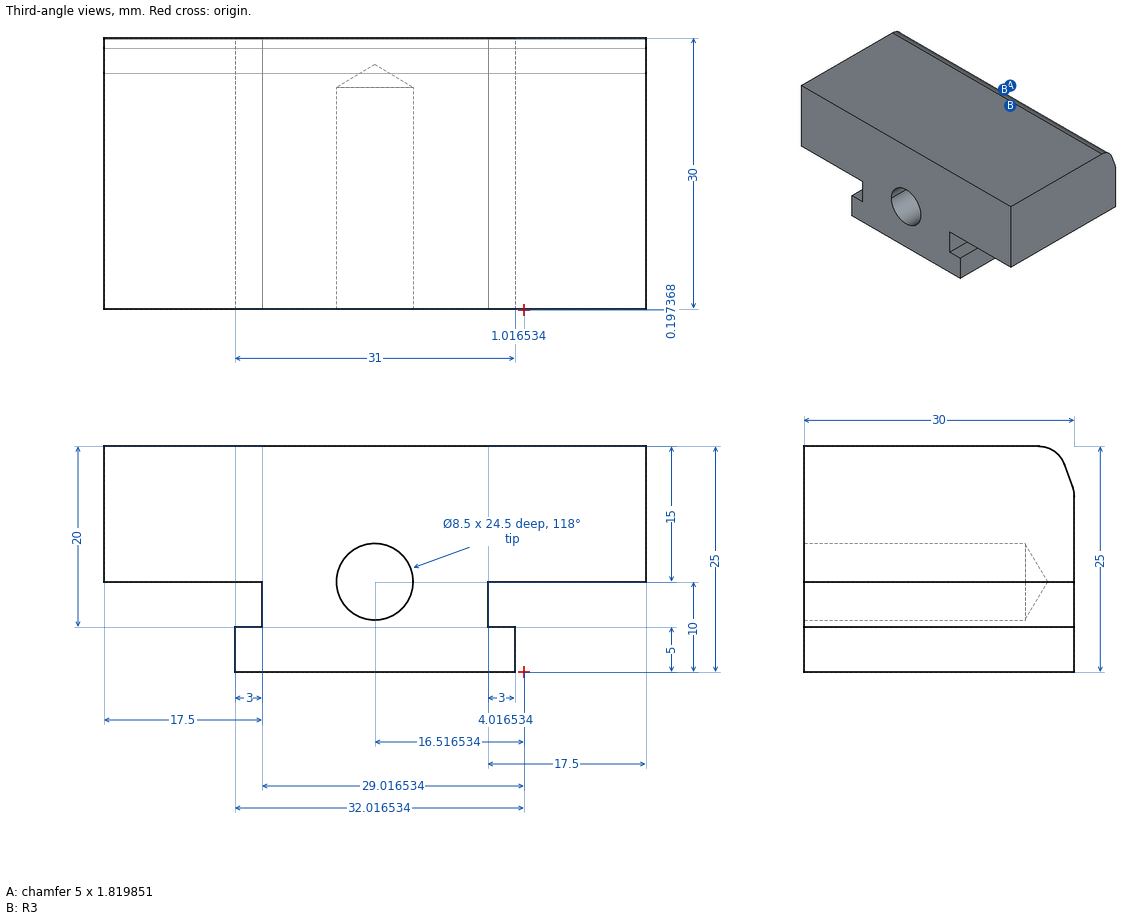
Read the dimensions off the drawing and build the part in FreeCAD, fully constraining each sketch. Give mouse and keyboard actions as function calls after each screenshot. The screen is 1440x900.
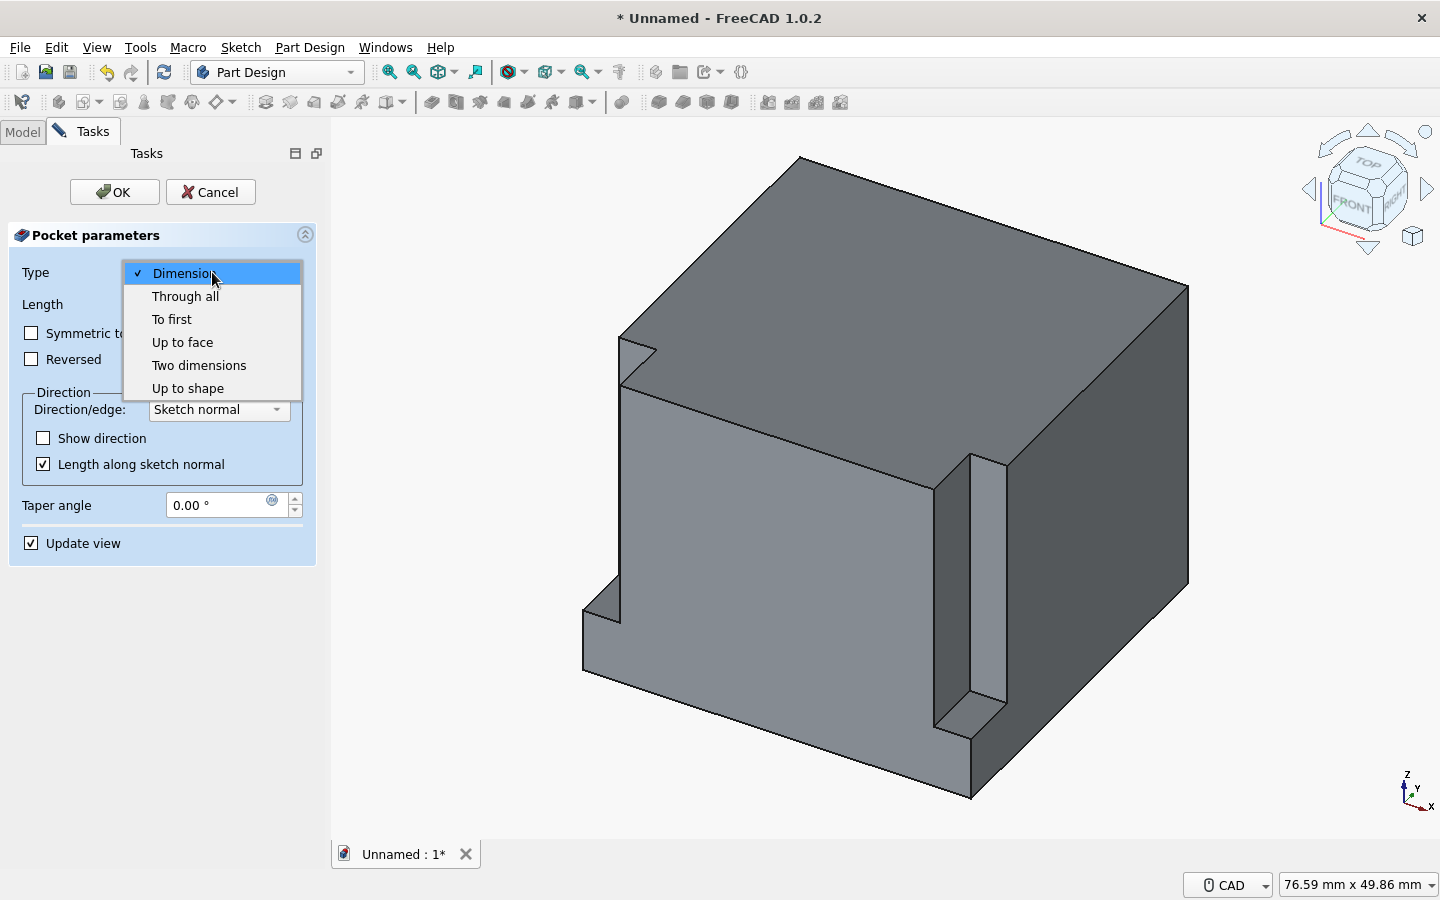
click(212, 296)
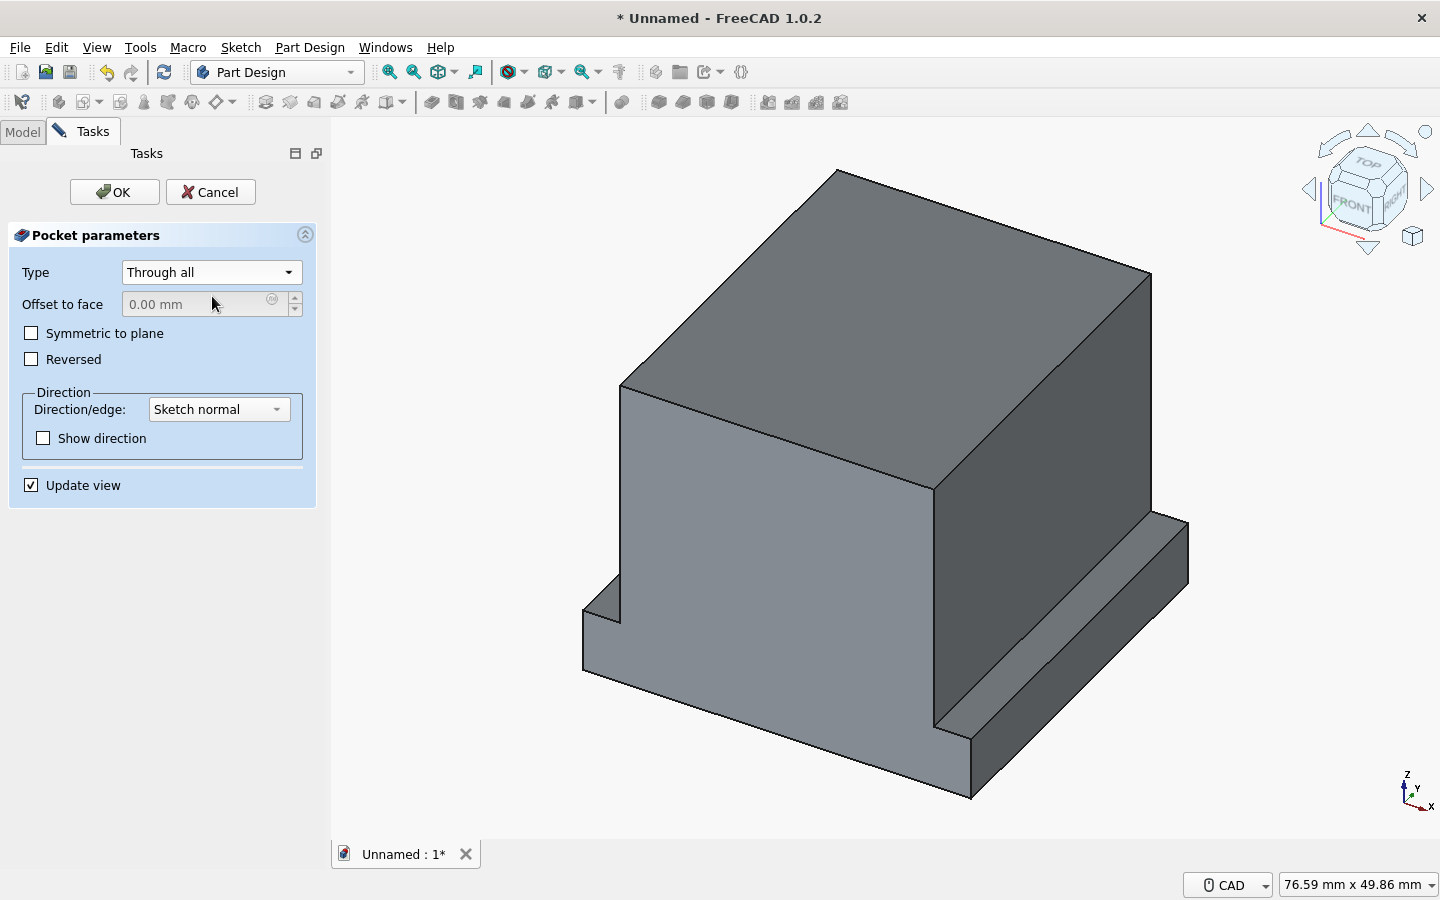
click(115, 192)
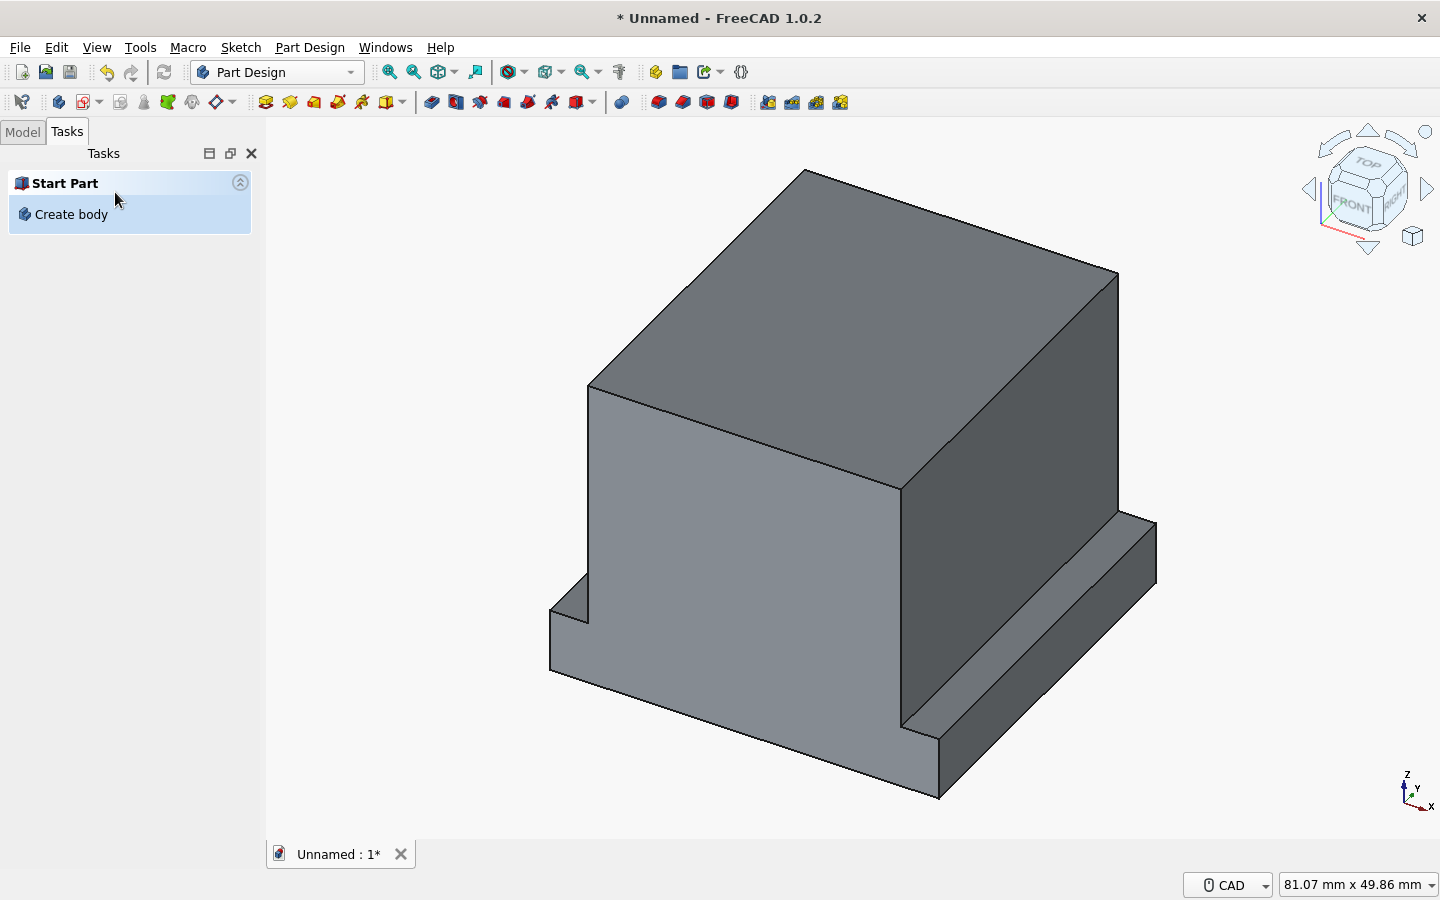
key(4)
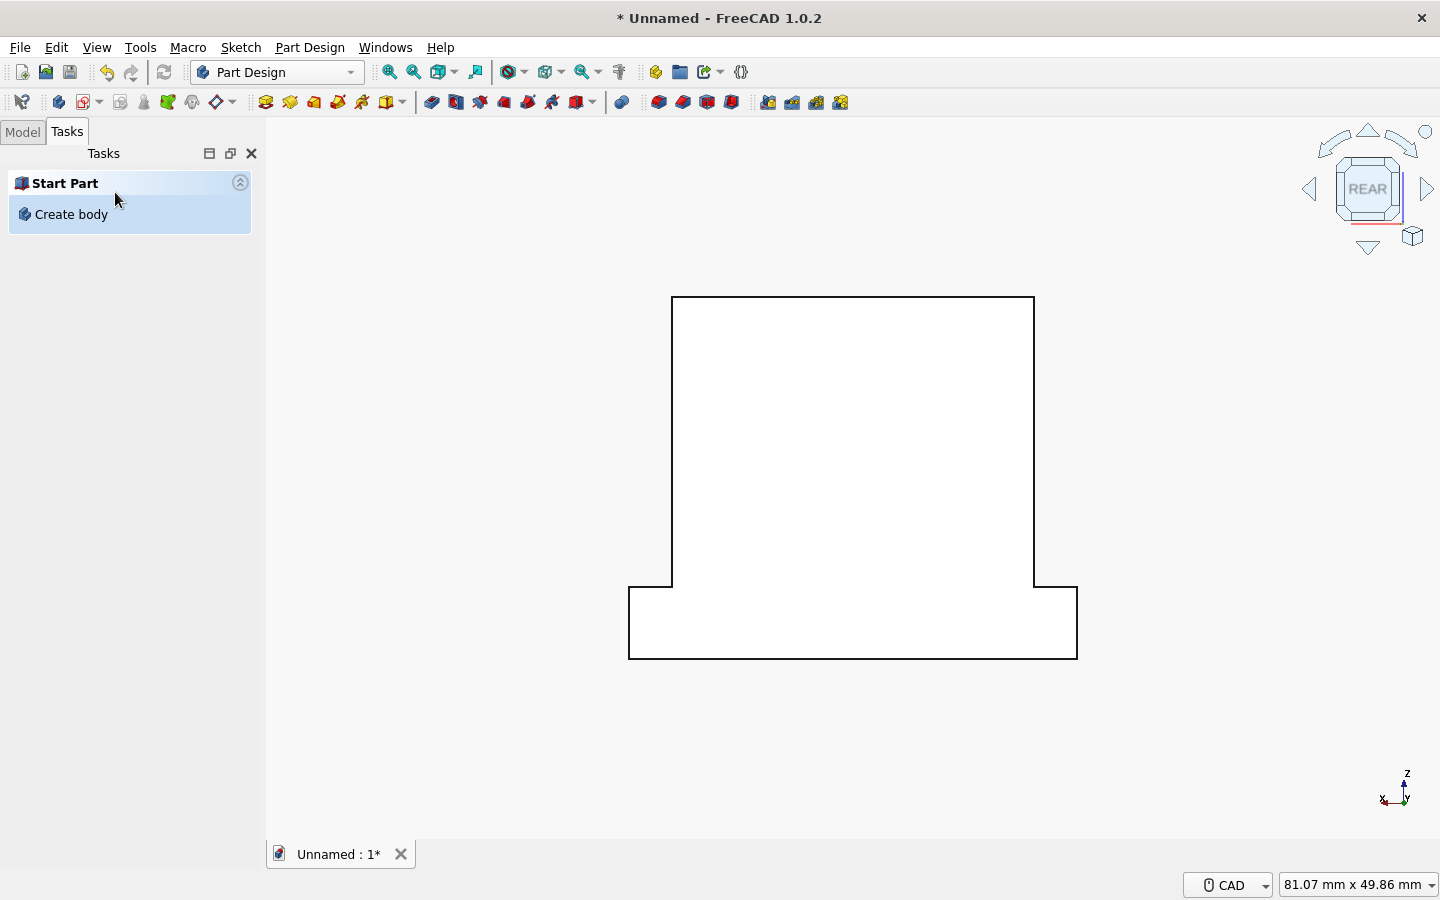
click(853, 477)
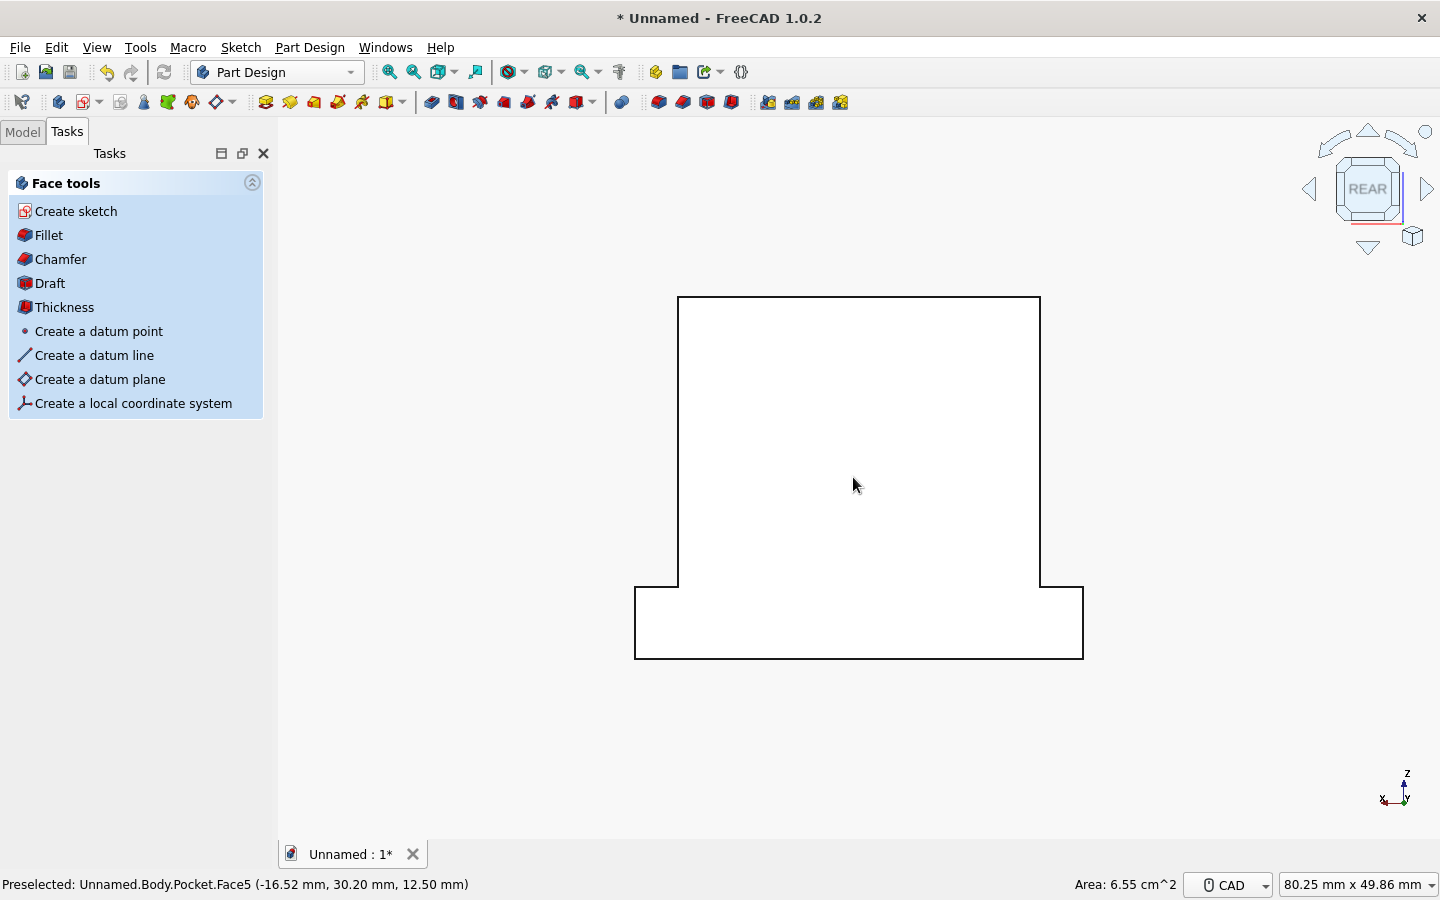
click(84, 102)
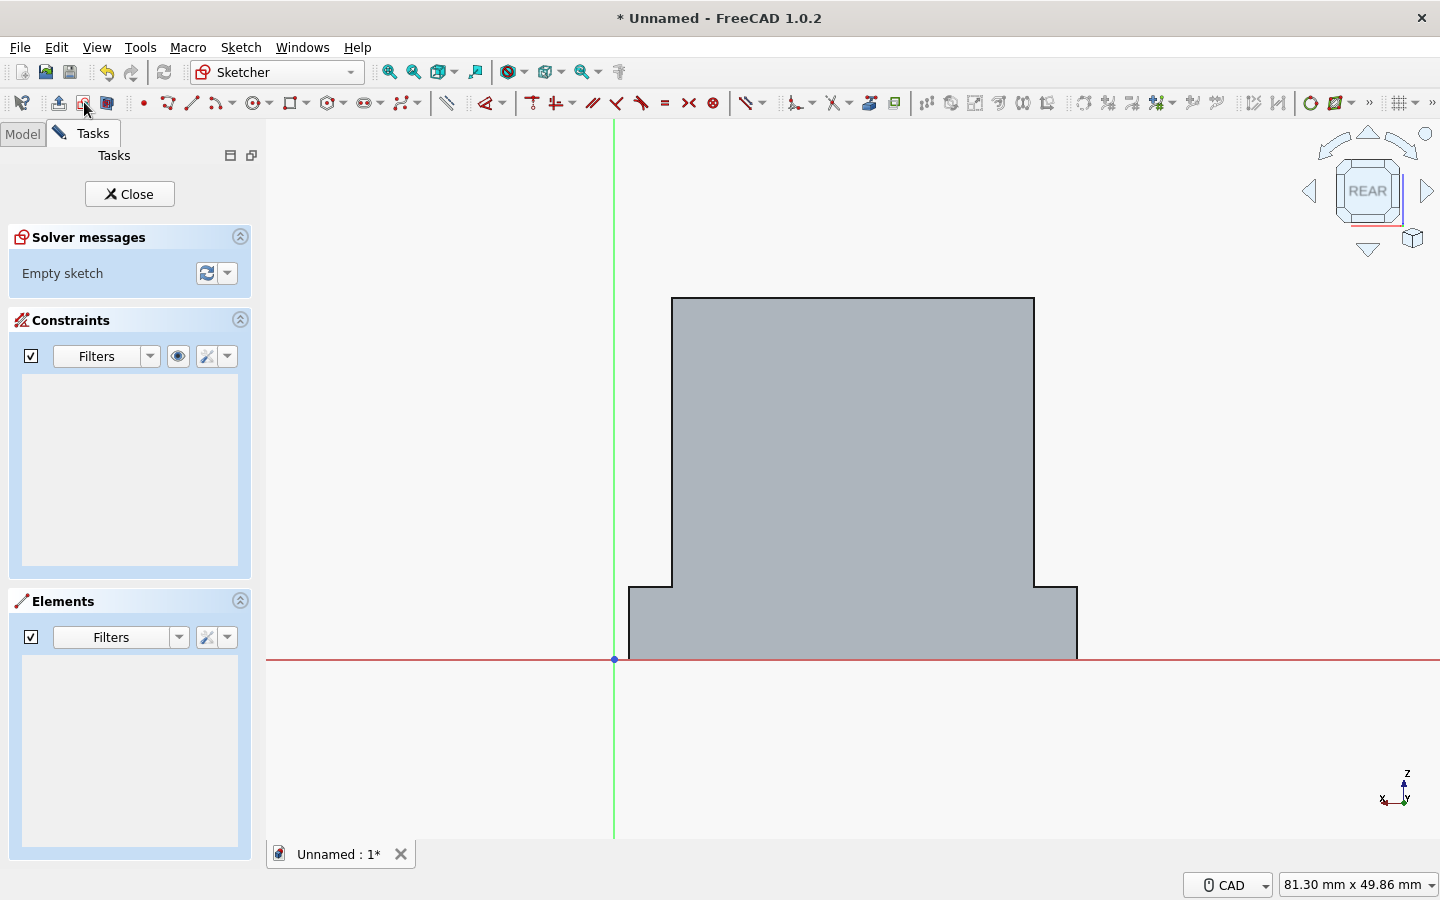
scroll(475, 479, down, 1)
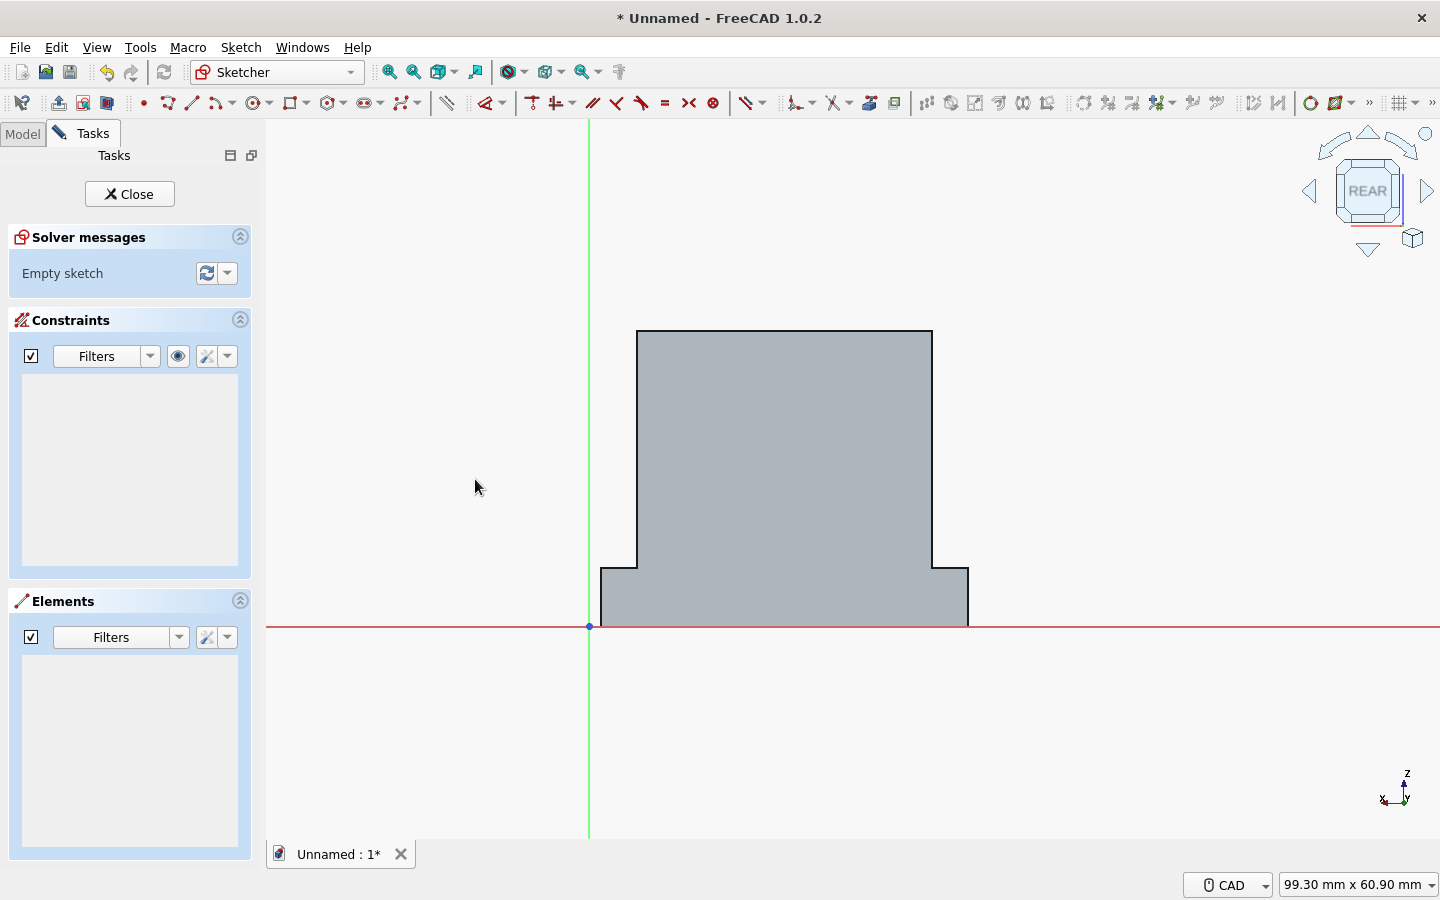
click(290, 104)